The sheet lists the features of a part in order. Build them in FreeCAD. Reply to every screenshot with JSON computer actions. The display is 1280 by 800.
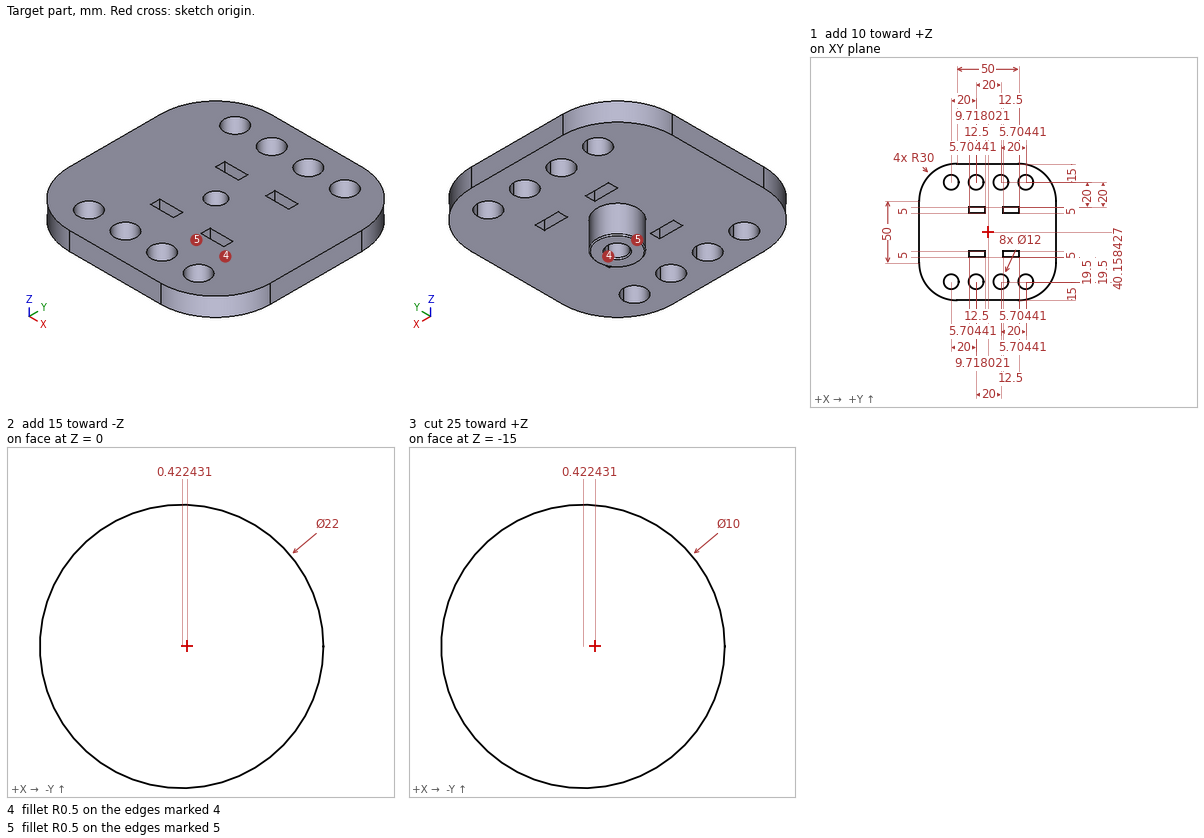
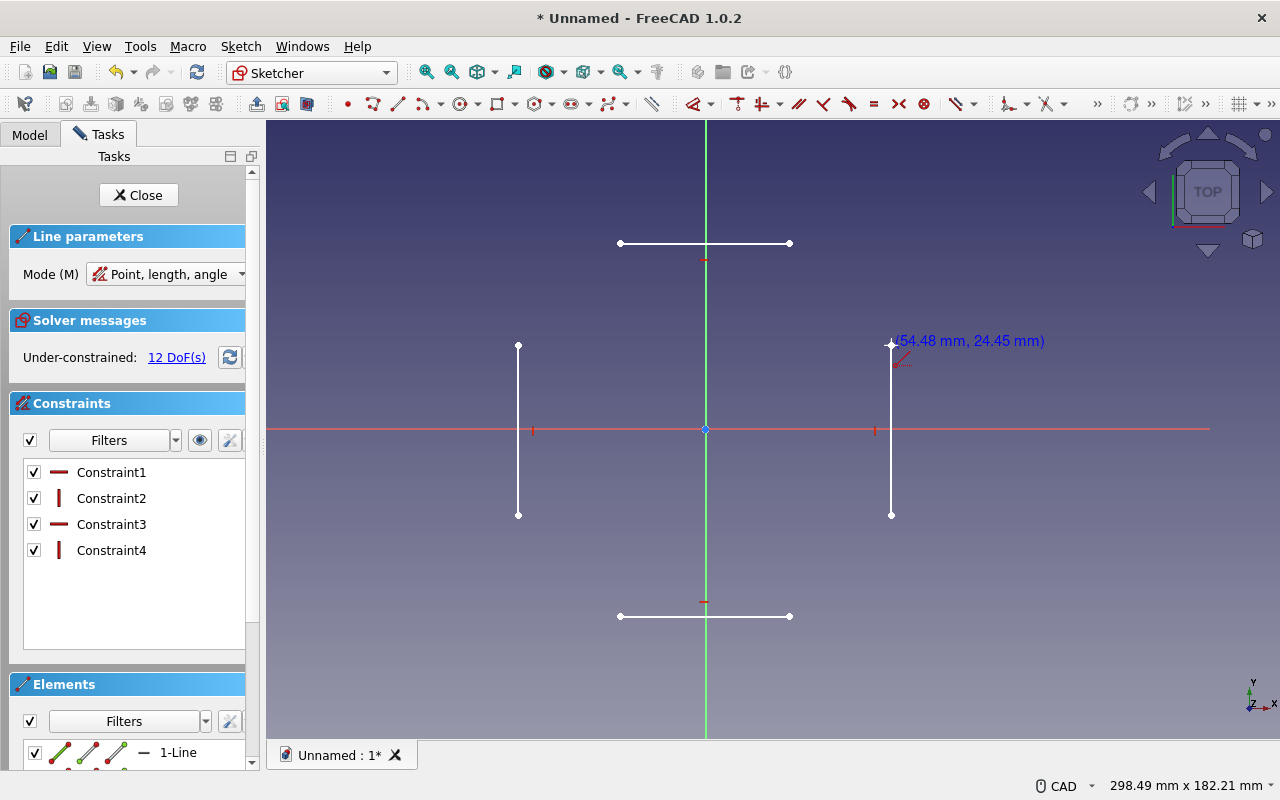
{"action": "left_click", "coordinate": [440, 104]}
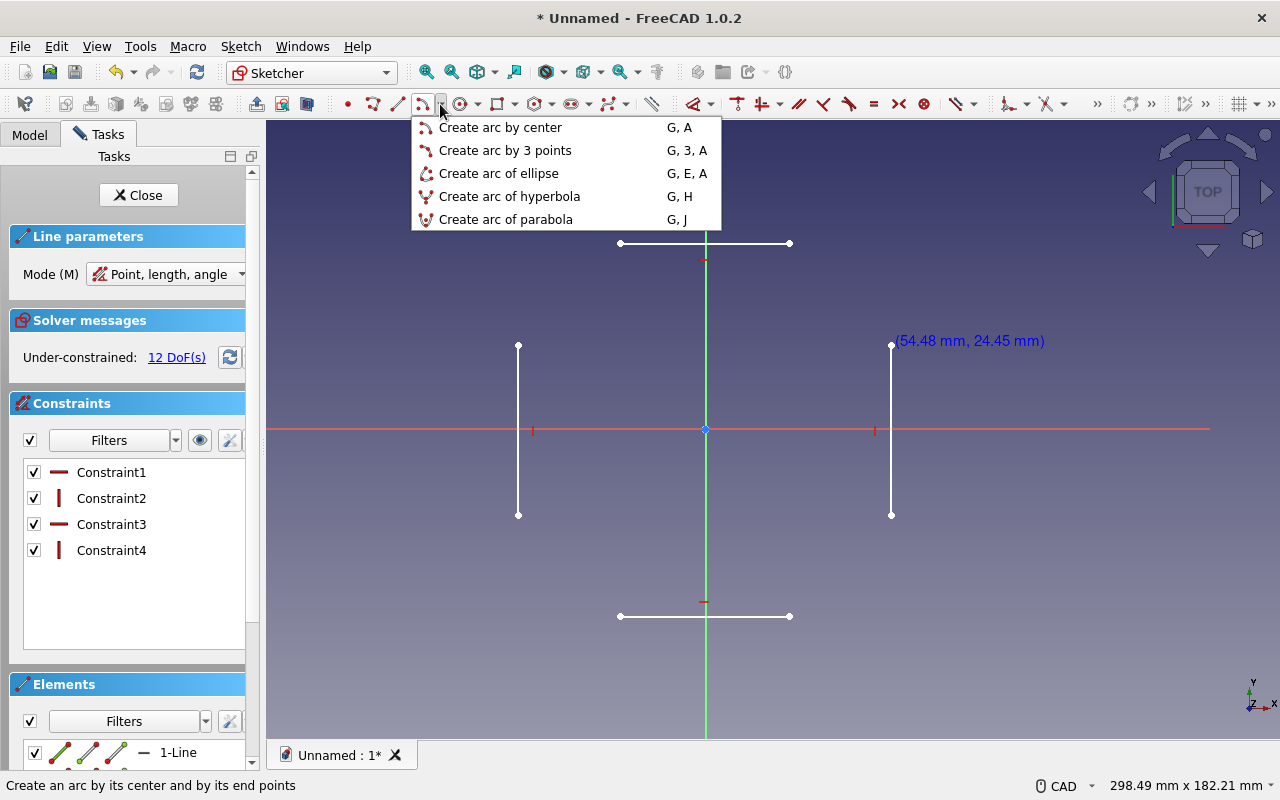
{"action": "left_click", "coordinate": [566, 150]}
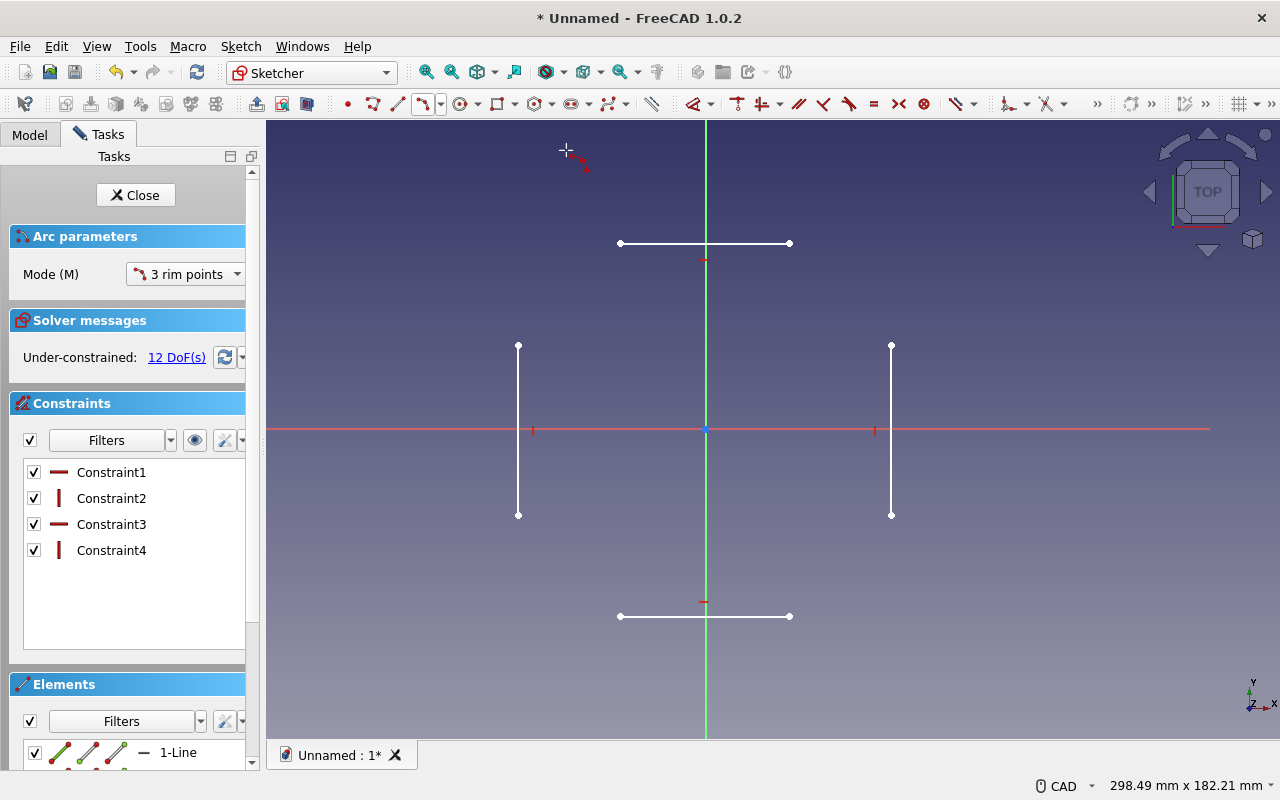
{"action": "left_click", "coordinate": [620, 244]}
{"action": "left_click", "coordinate": [518, 346]}
{"action": "left_click", "coordinate": [548, 273]}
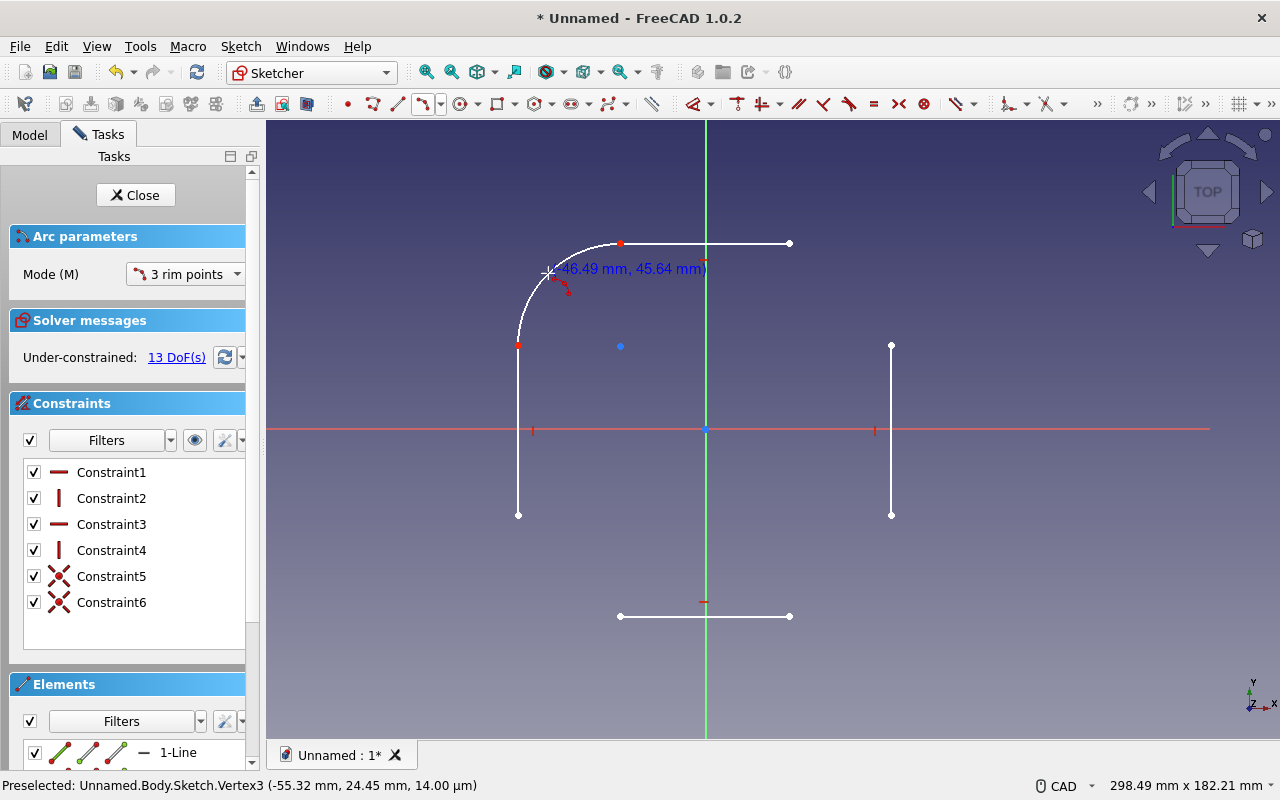
{"action": "left_click", "coordinate": [518, 516]}
{"action": "left_click", "coordinate": [620, 617]}
{"action": "left_click", "coordinate": [548, 587]}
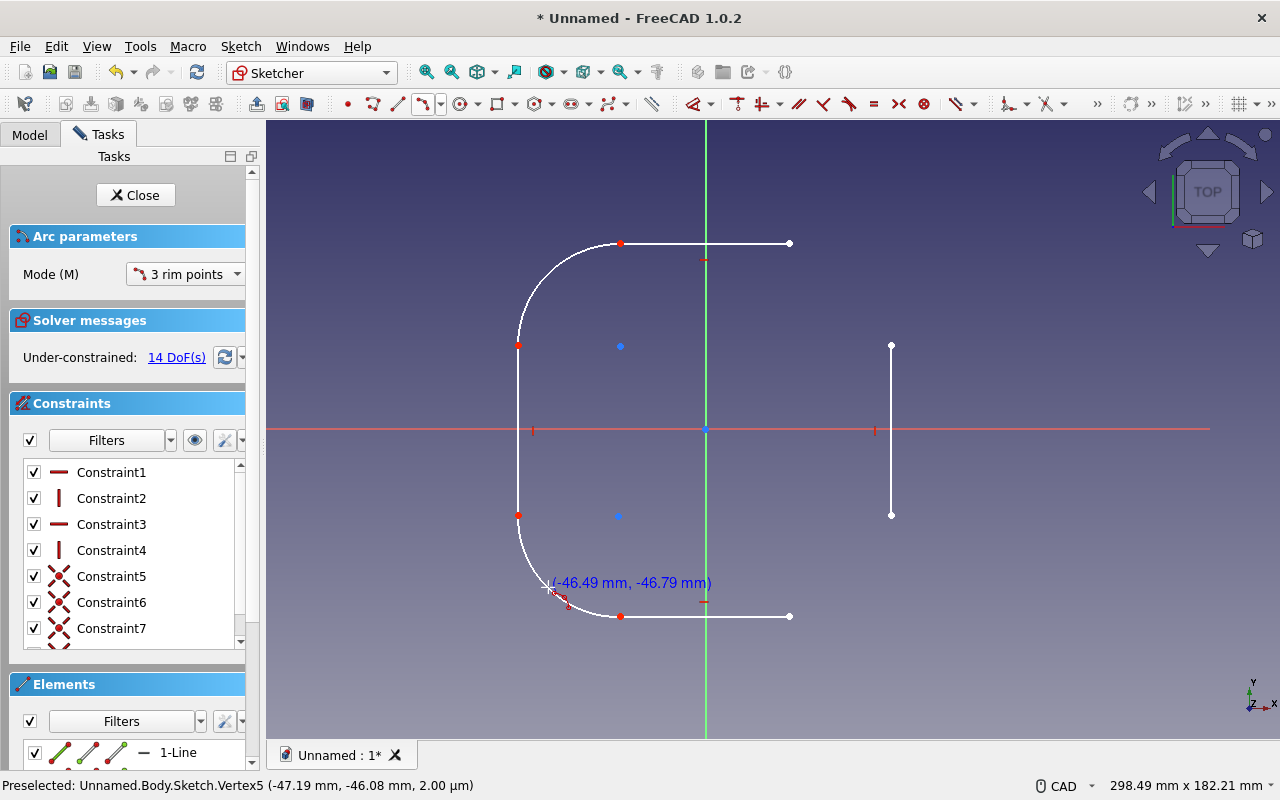
{"action": "left_click", "coordinate": [789, 617]}
{"action": "left_click", "coordinate": [891, 516]}
{"action": "left_click", "coordinate": [861, 587]}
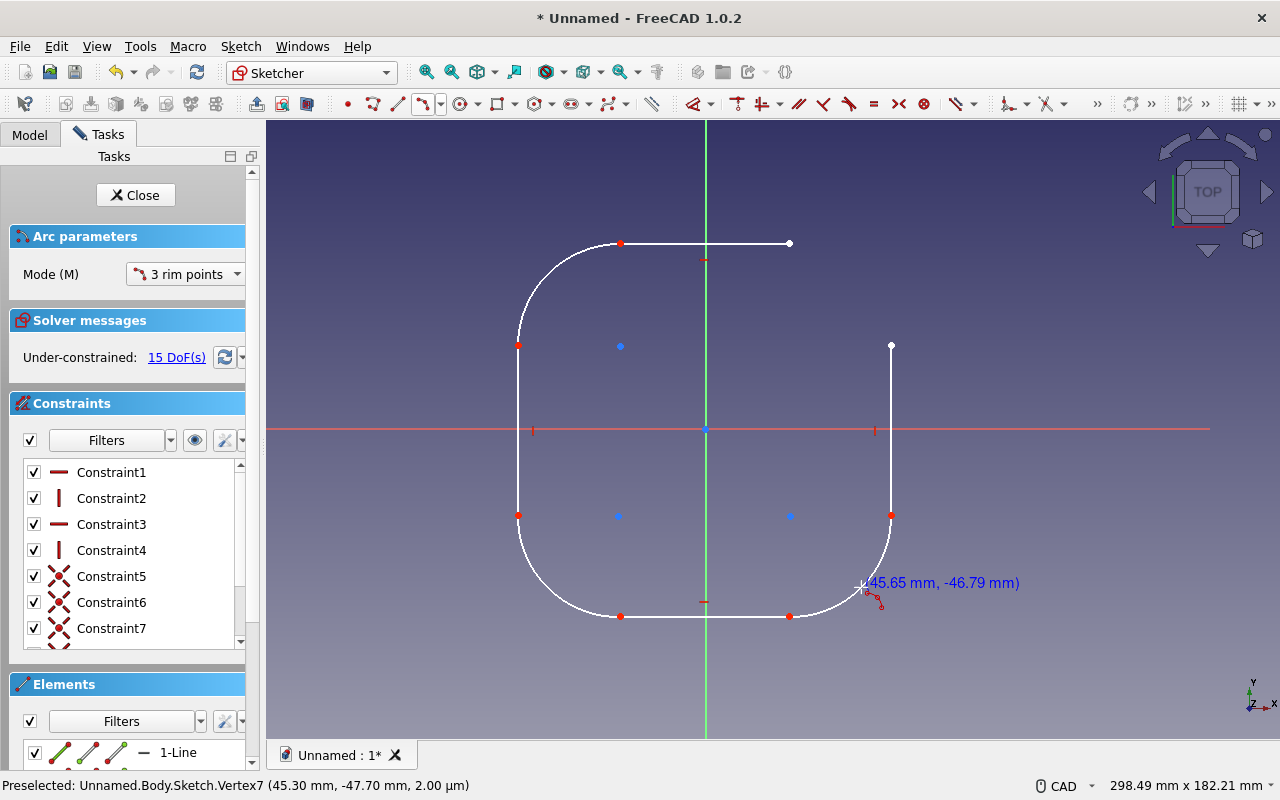
{"action": "left_click", "coordinate": [891, 346]}
{"action": "left_click", "coordinate": [789, 244]}
{"action": "left_click", "coordinate": [861, 273]}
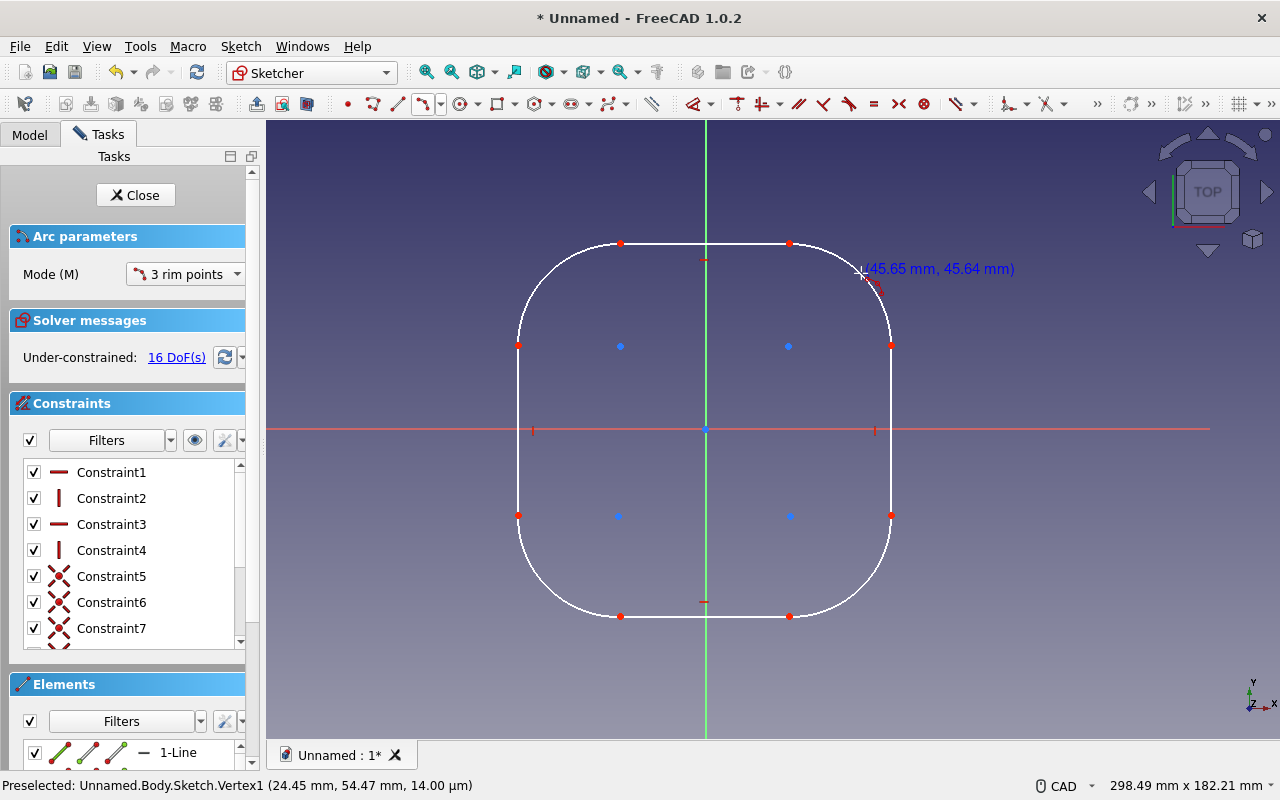
{"action": "left_click", "coordinate": [496, 104]}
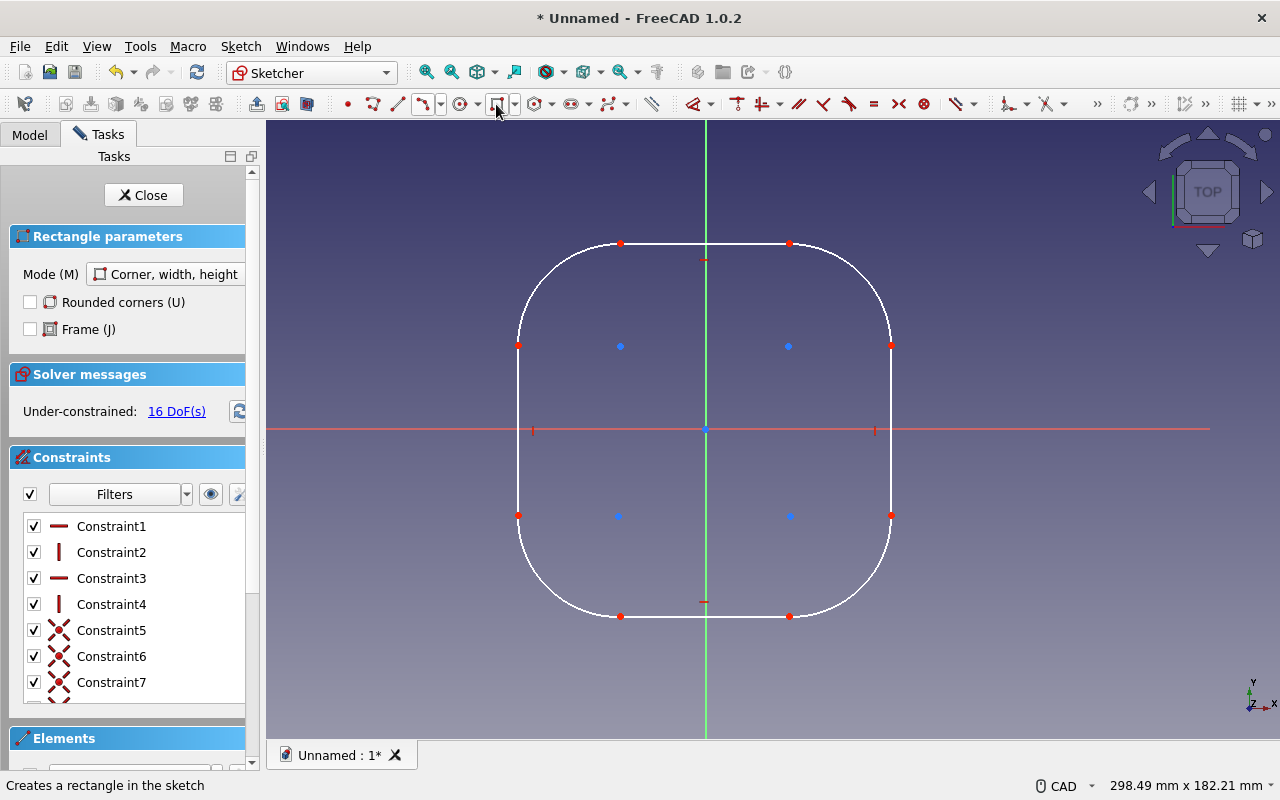
{"action": "left_click", "coordinate": [747, 482]}
{"action": "mouse_move", "coordinate": [789, 499]}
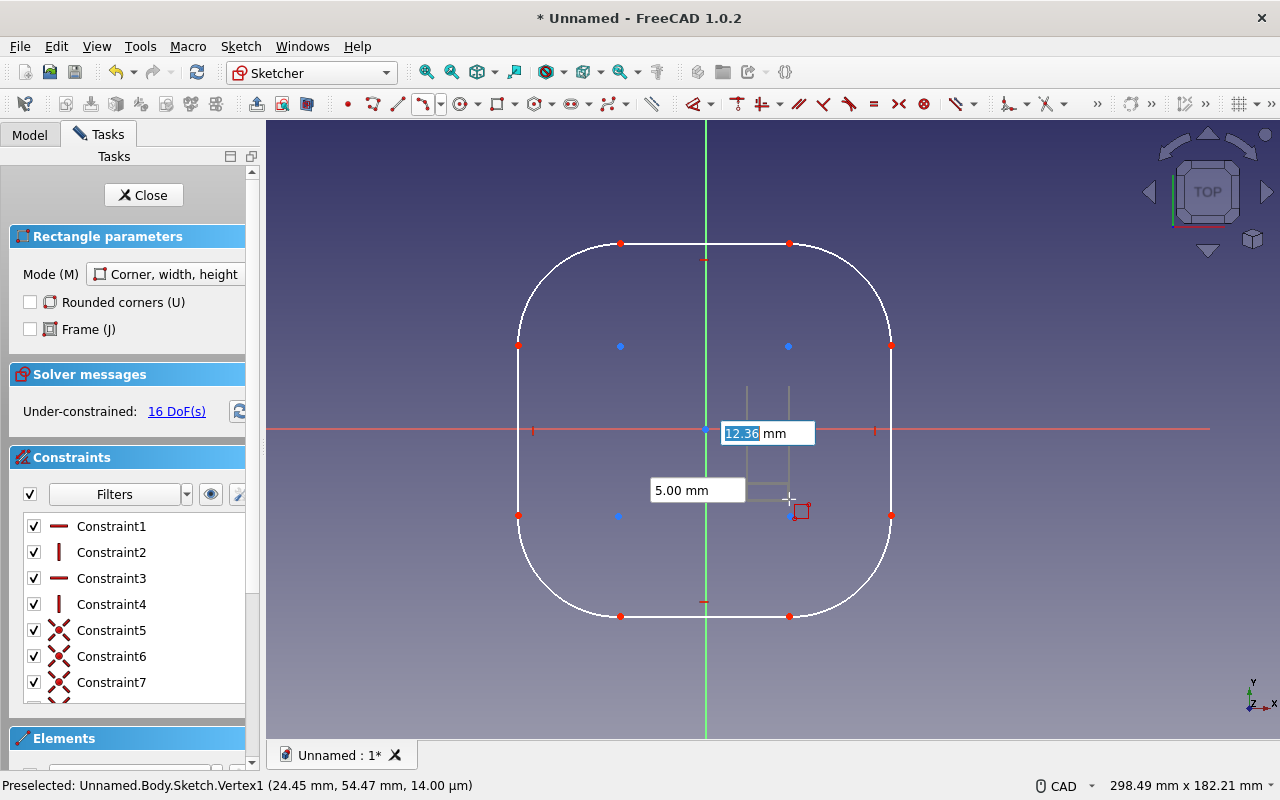
{"action": "type", "text": "12.5"}
{"action": "key", "text": "Tab"}
{"action": "type", "text": "5"}
{"action": "key", "text": "Return"}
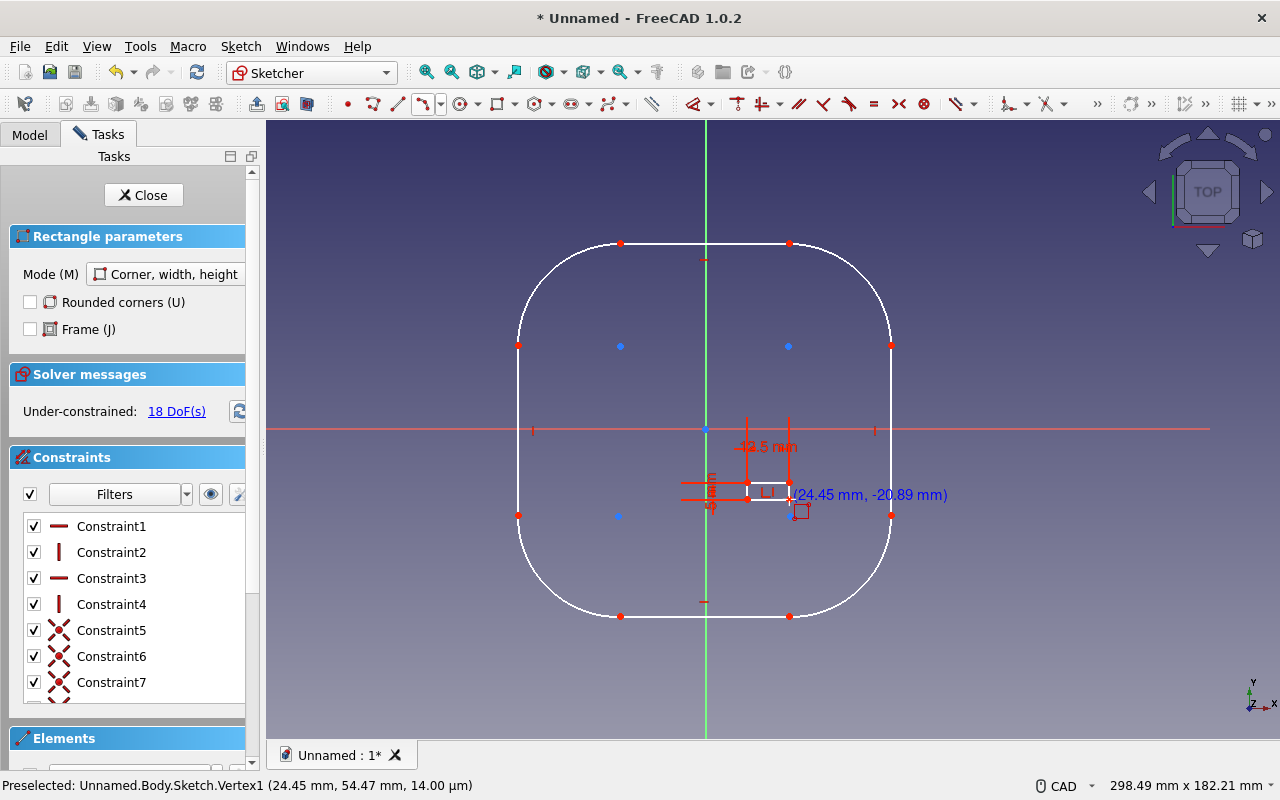
{"action": "left_click", "coordinate": [654, 482]}